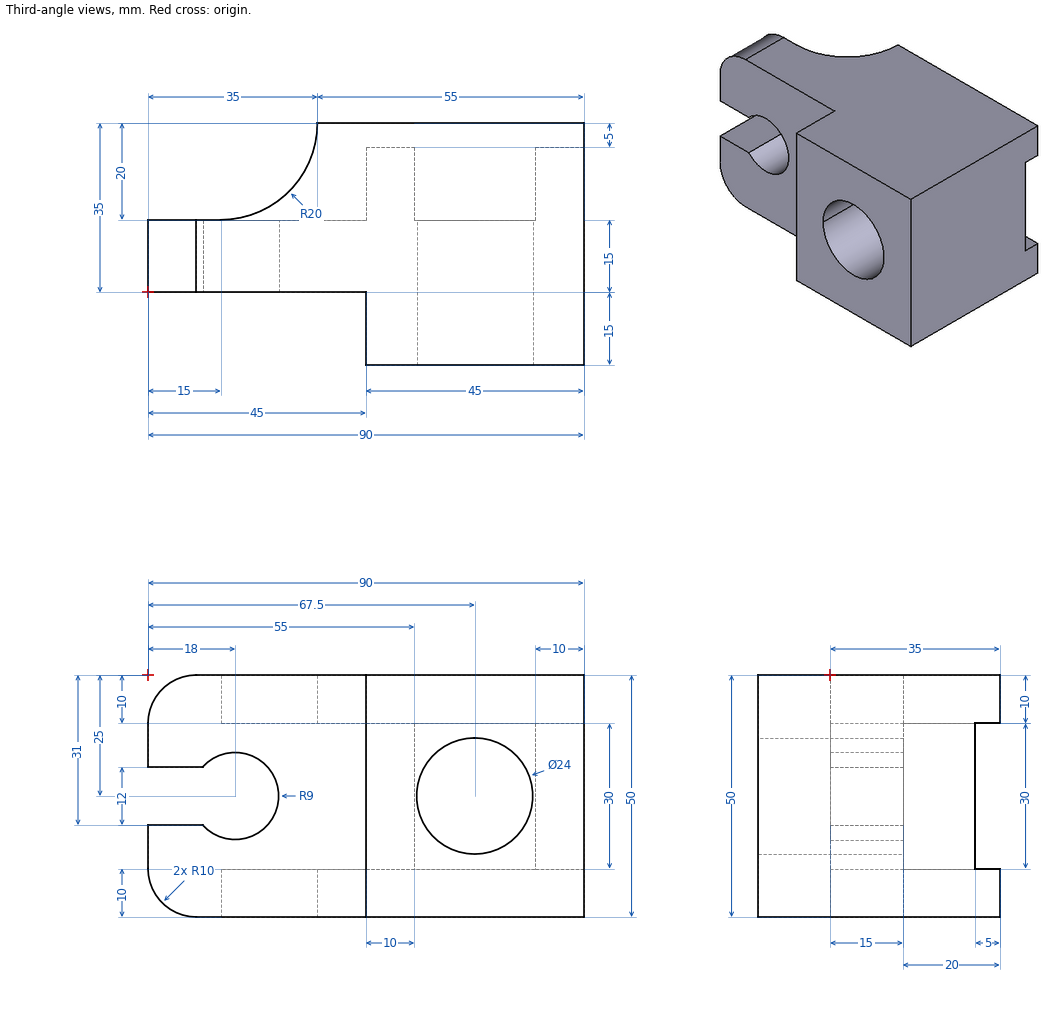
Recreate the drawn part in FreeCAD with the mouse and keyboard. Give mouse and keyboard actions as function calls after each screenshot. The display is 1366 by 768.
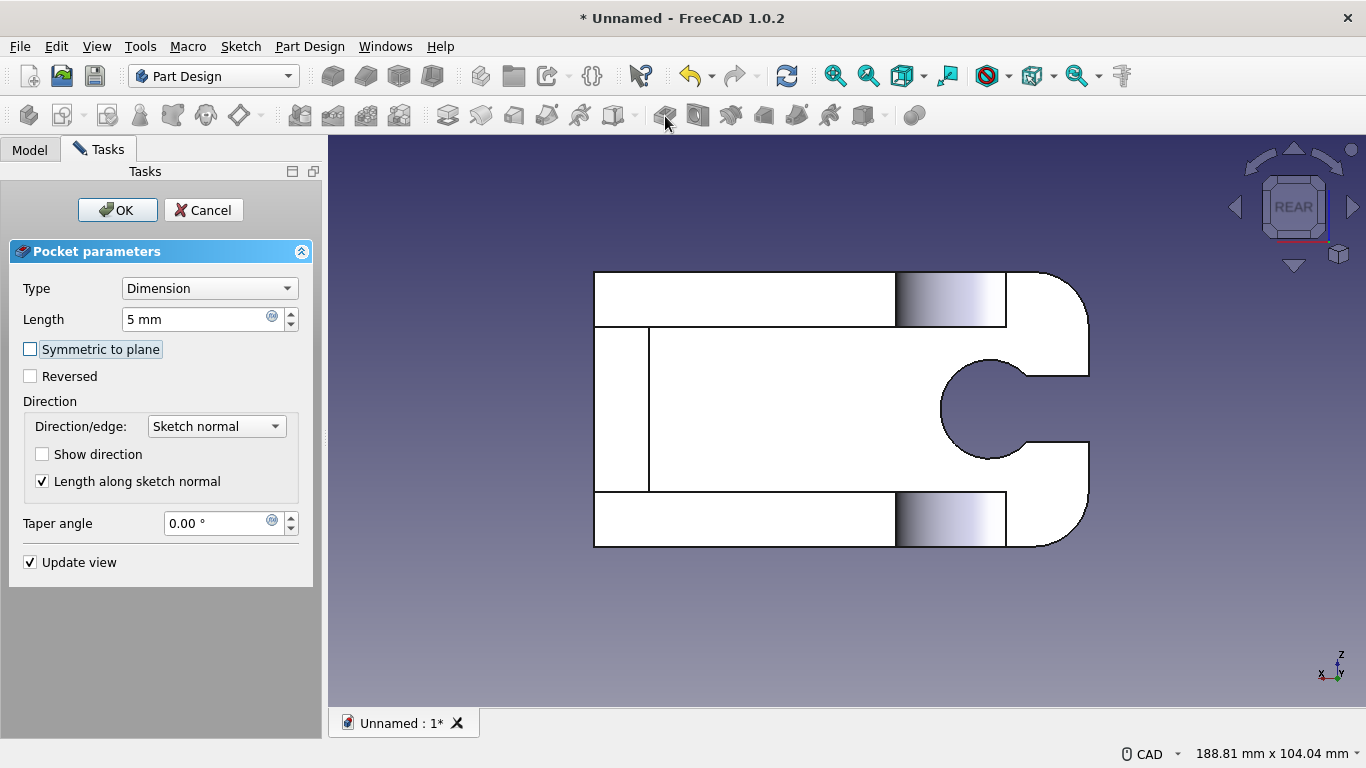
click(118, 210)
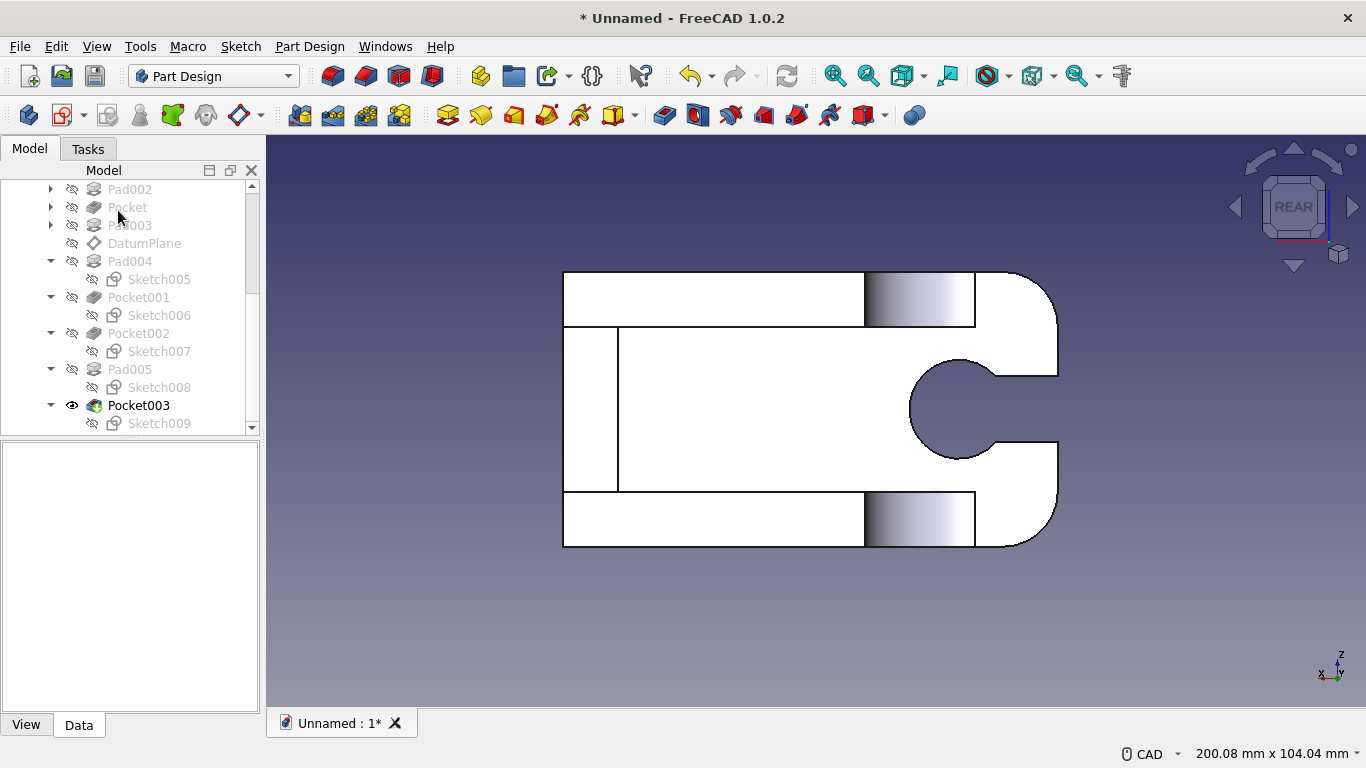
click(628, 518)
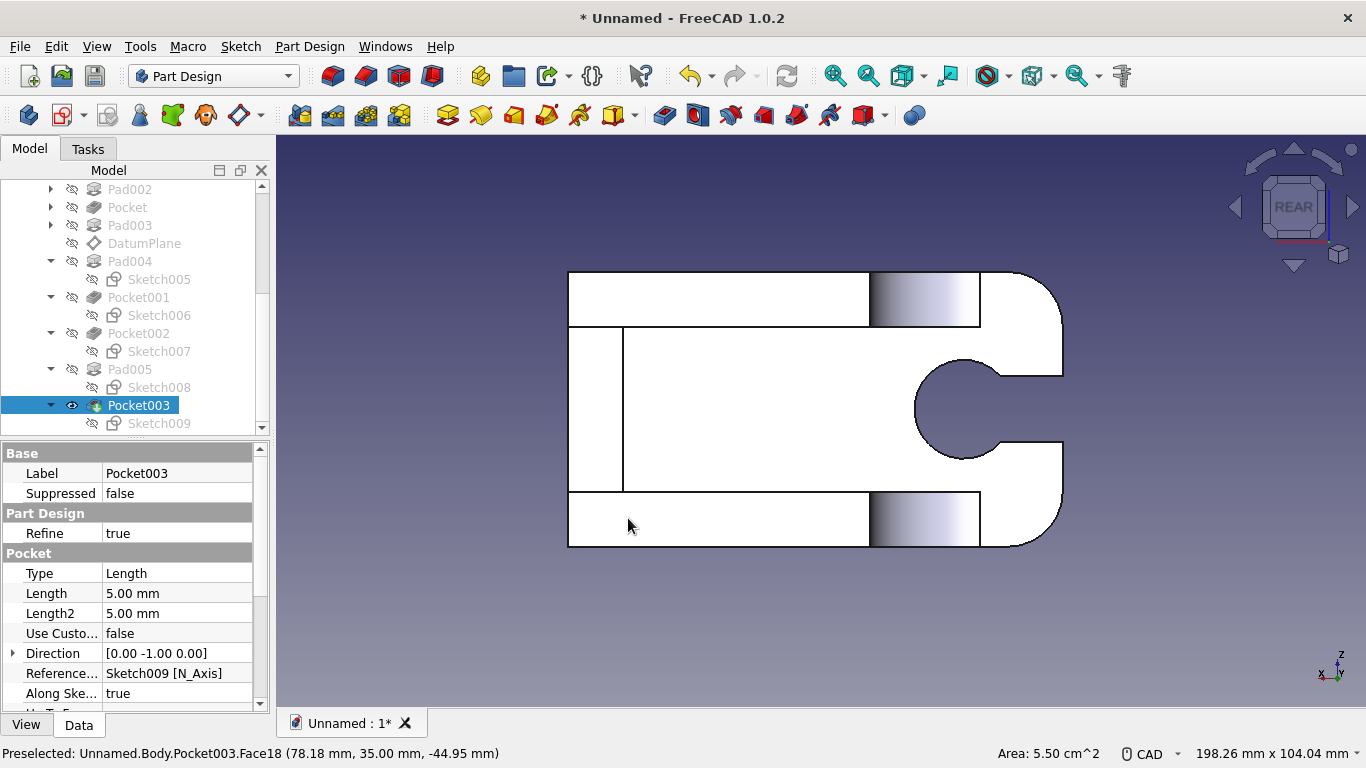
click(62, 116)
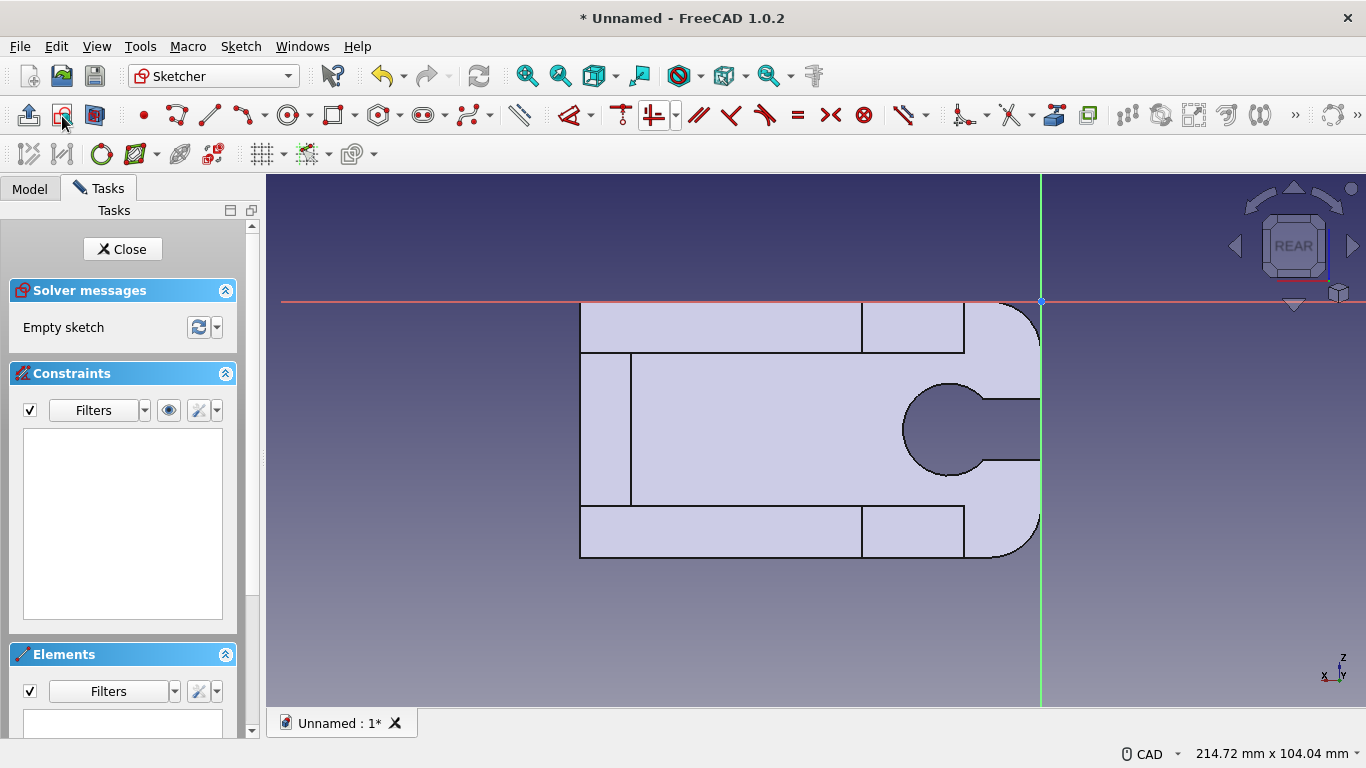
scroll(1201, 330, up, 2)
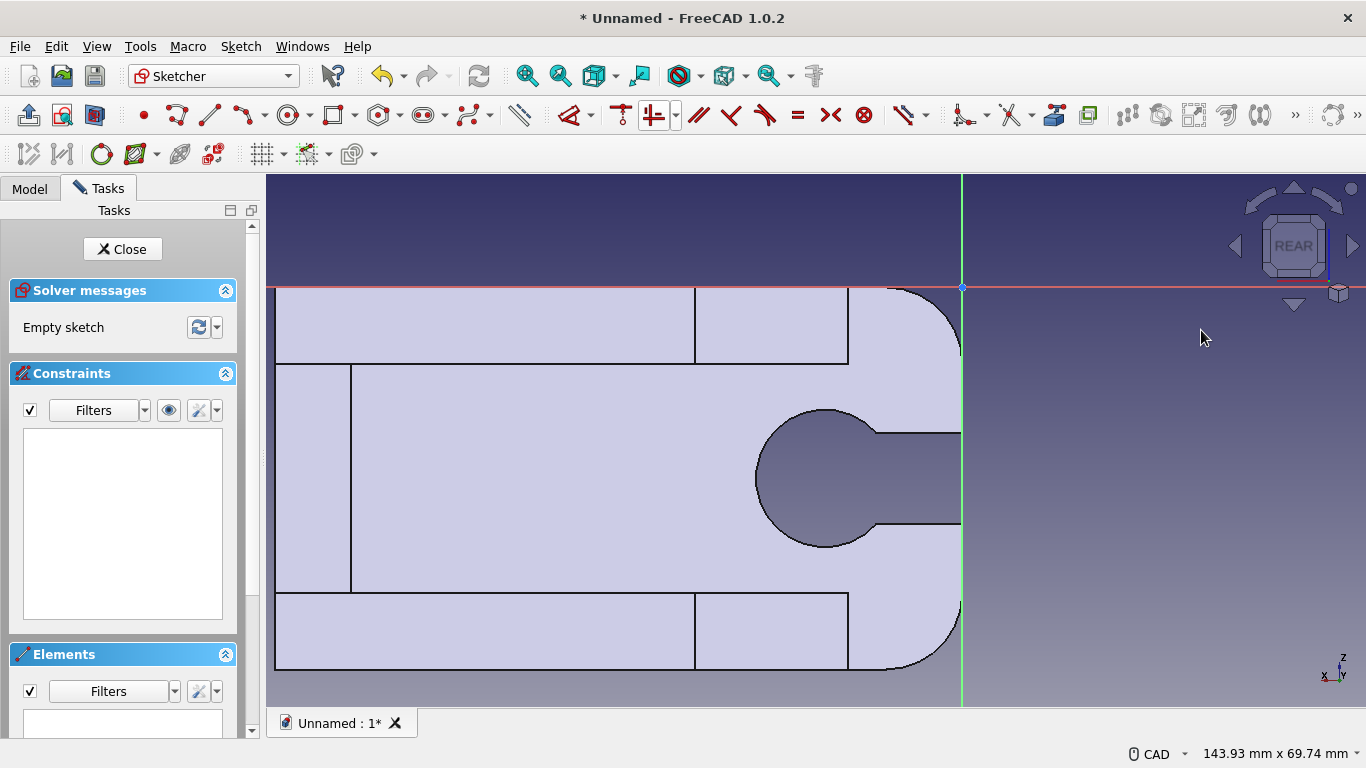
click(332, 116)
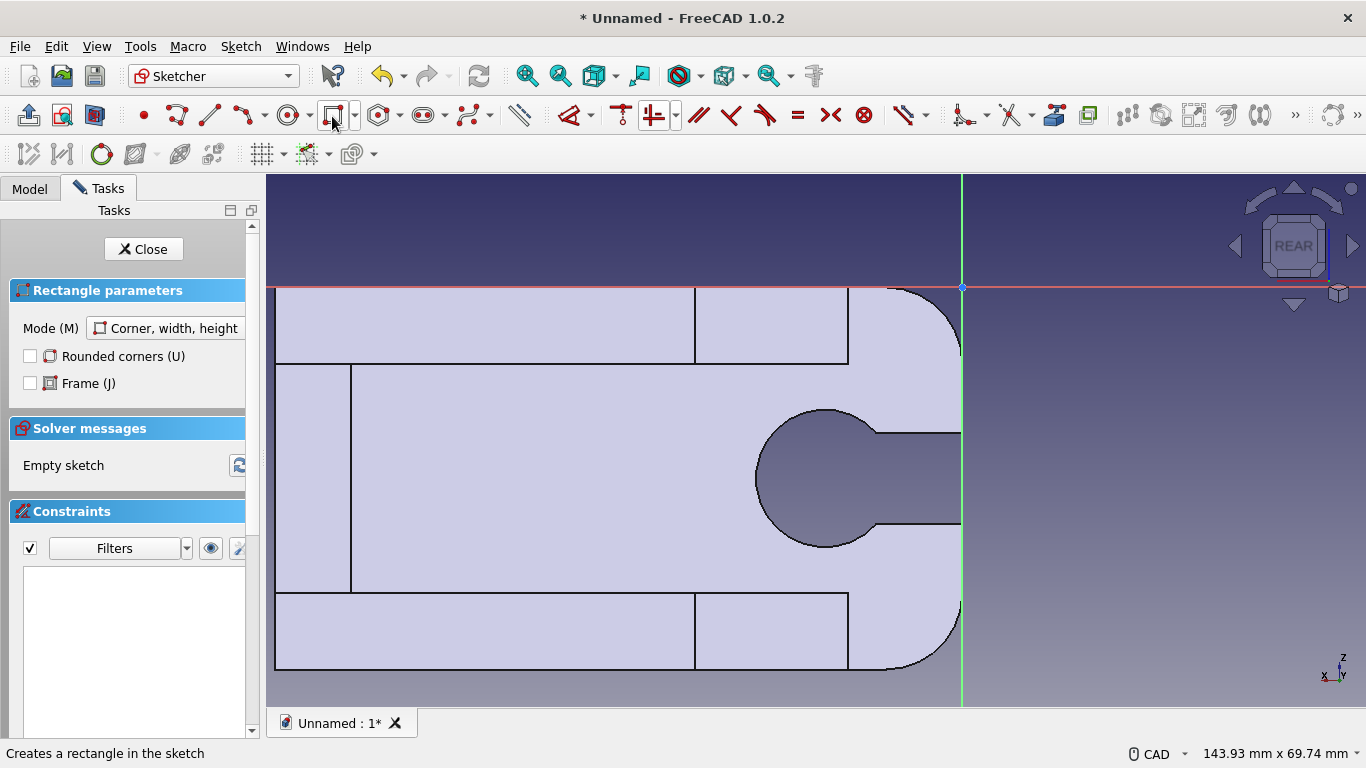
click(542, 364)
click(618, 593)
key(Escape)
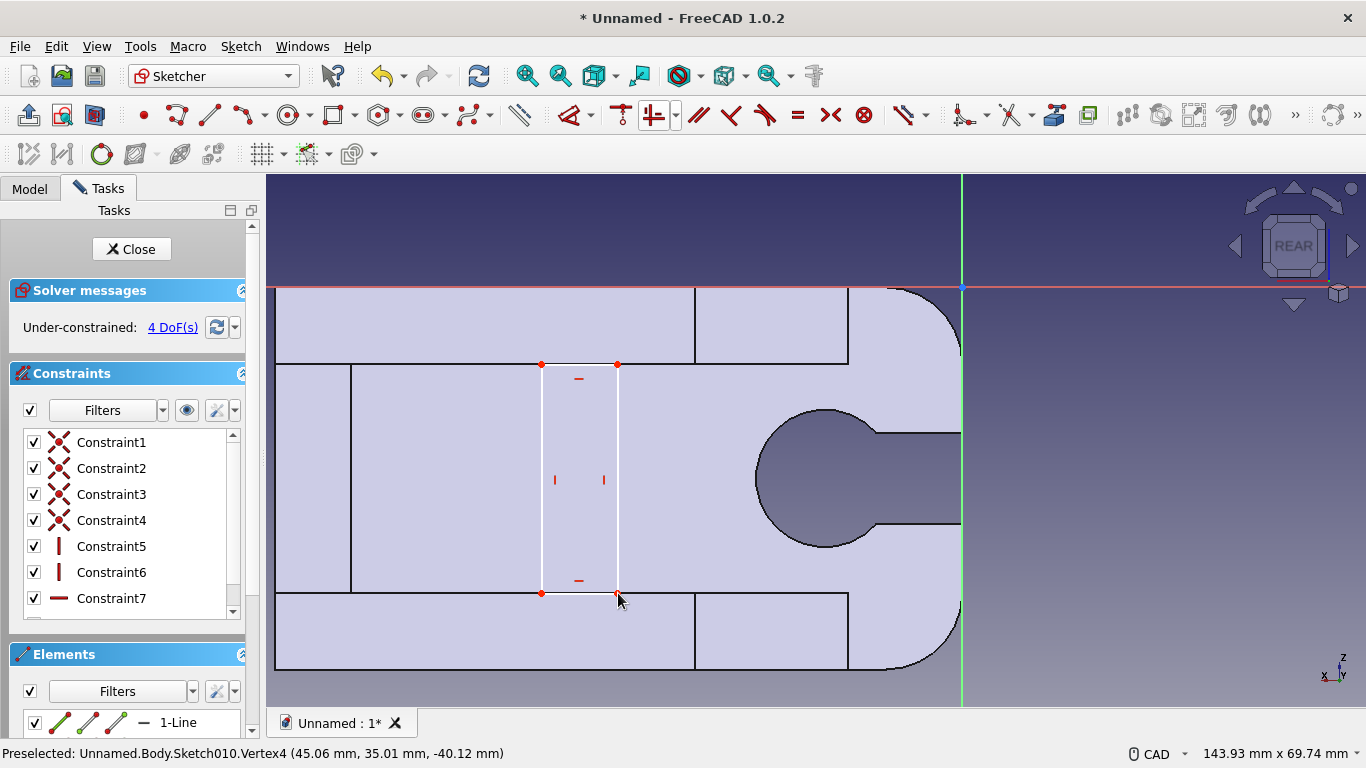
key(d)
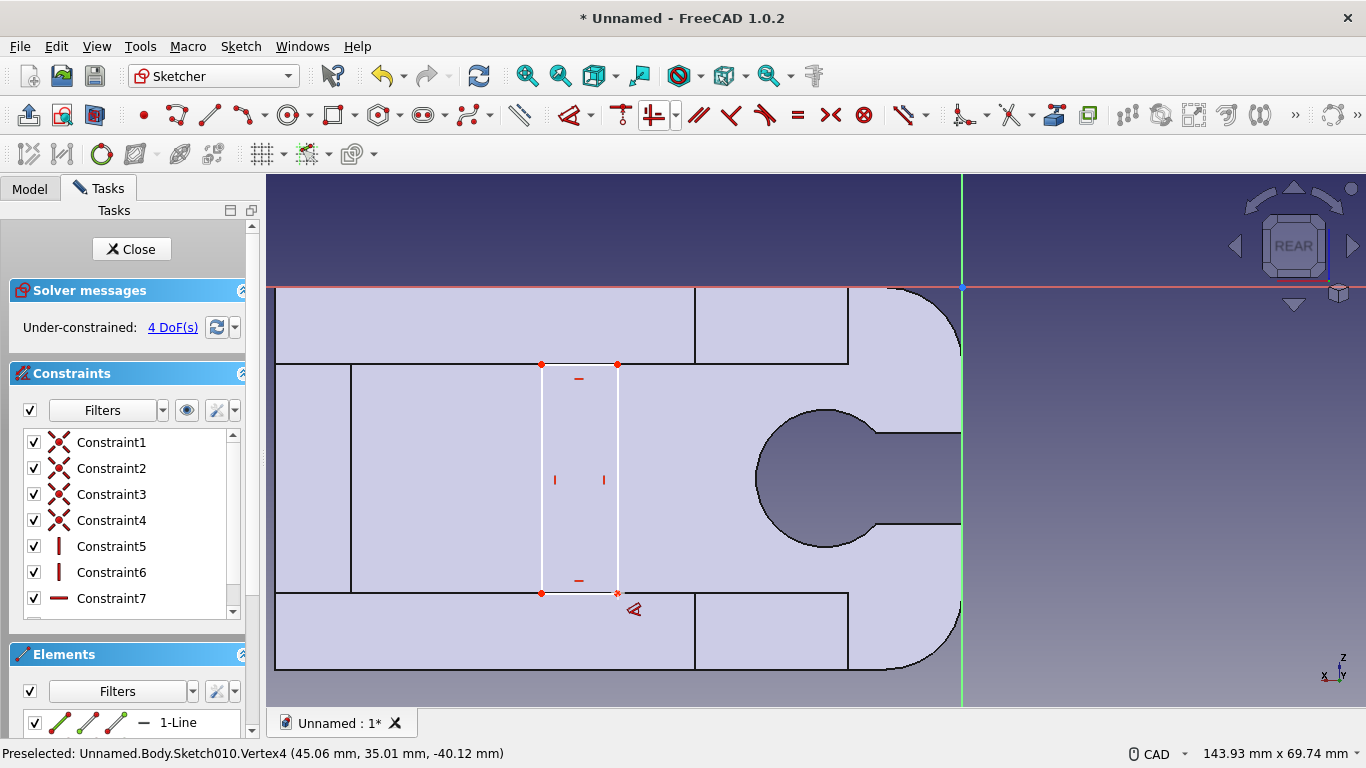
click(542, 434)
click(508, 480)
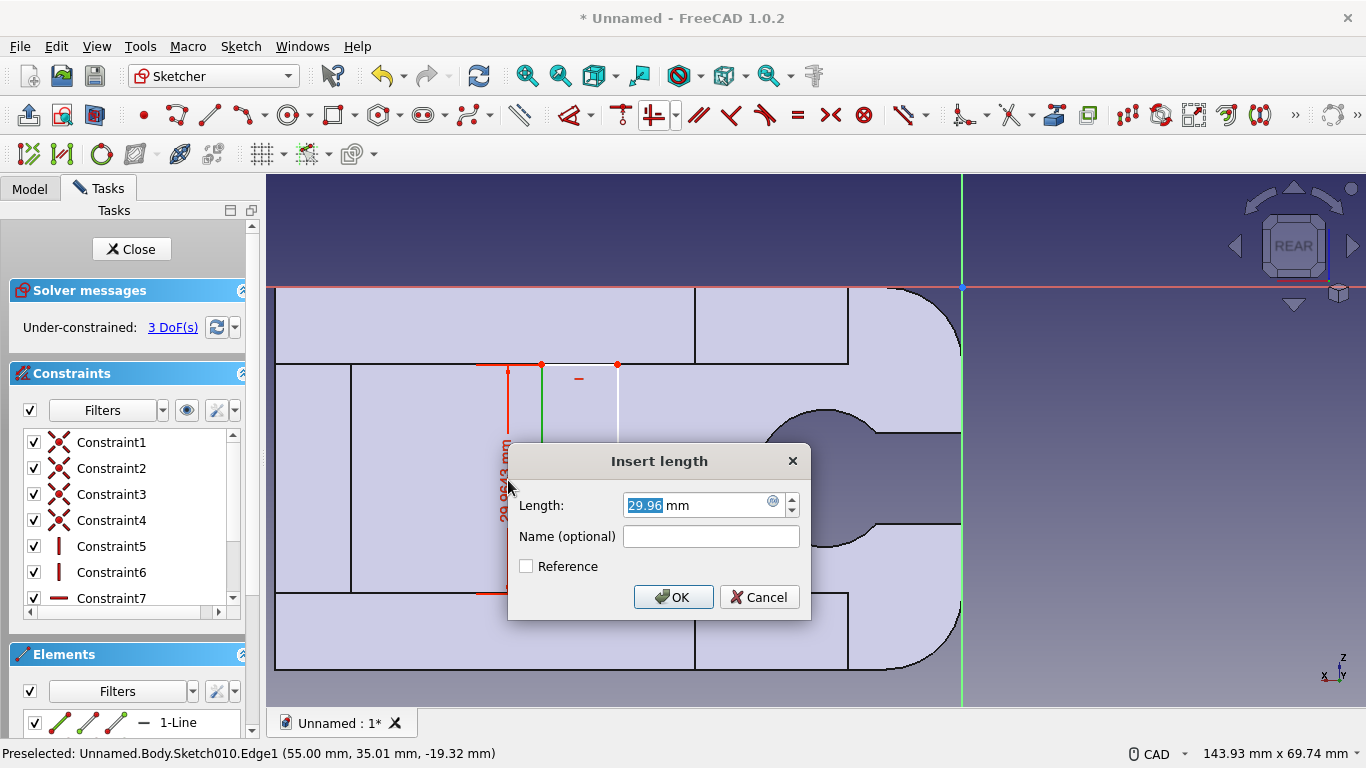
text(30)
key(Return)